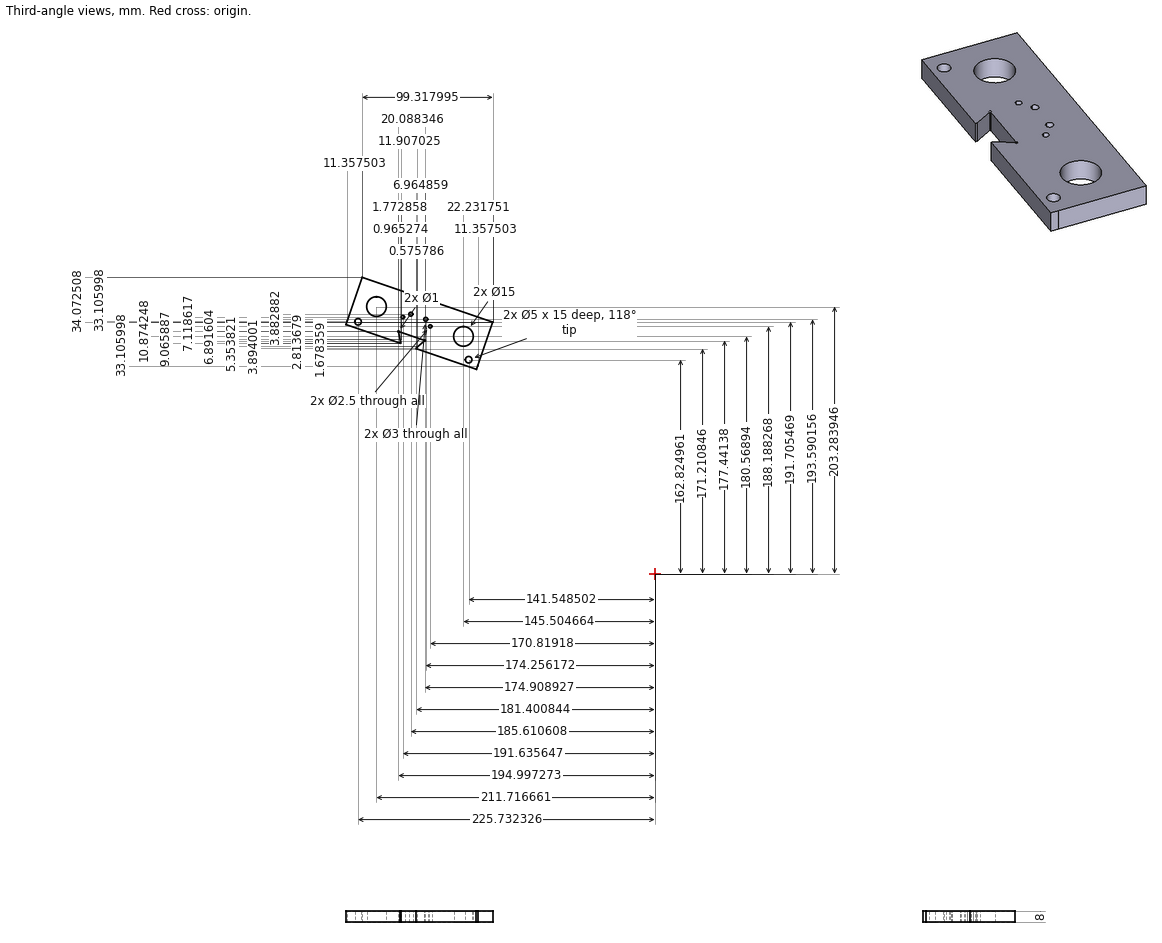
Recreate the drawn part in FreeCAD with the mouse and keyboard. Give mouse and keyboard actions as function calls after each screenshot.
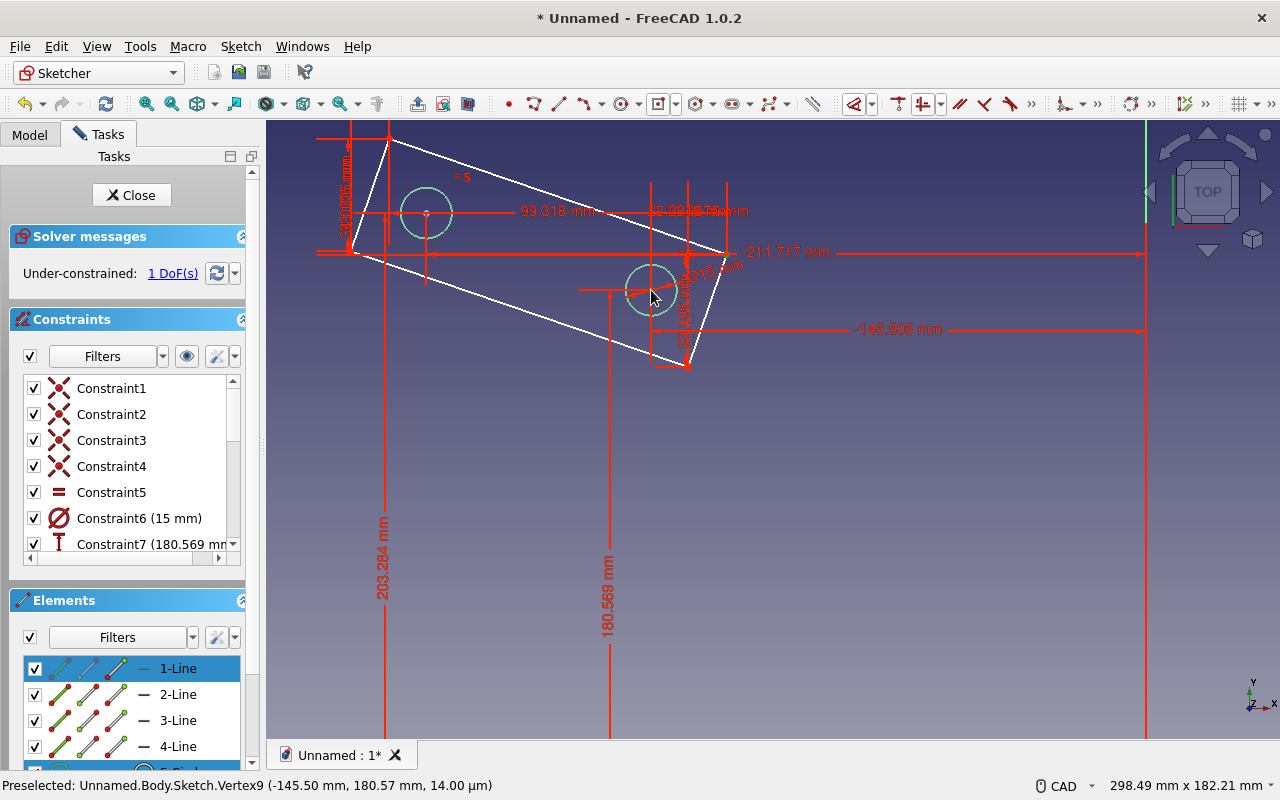
click(872, 104)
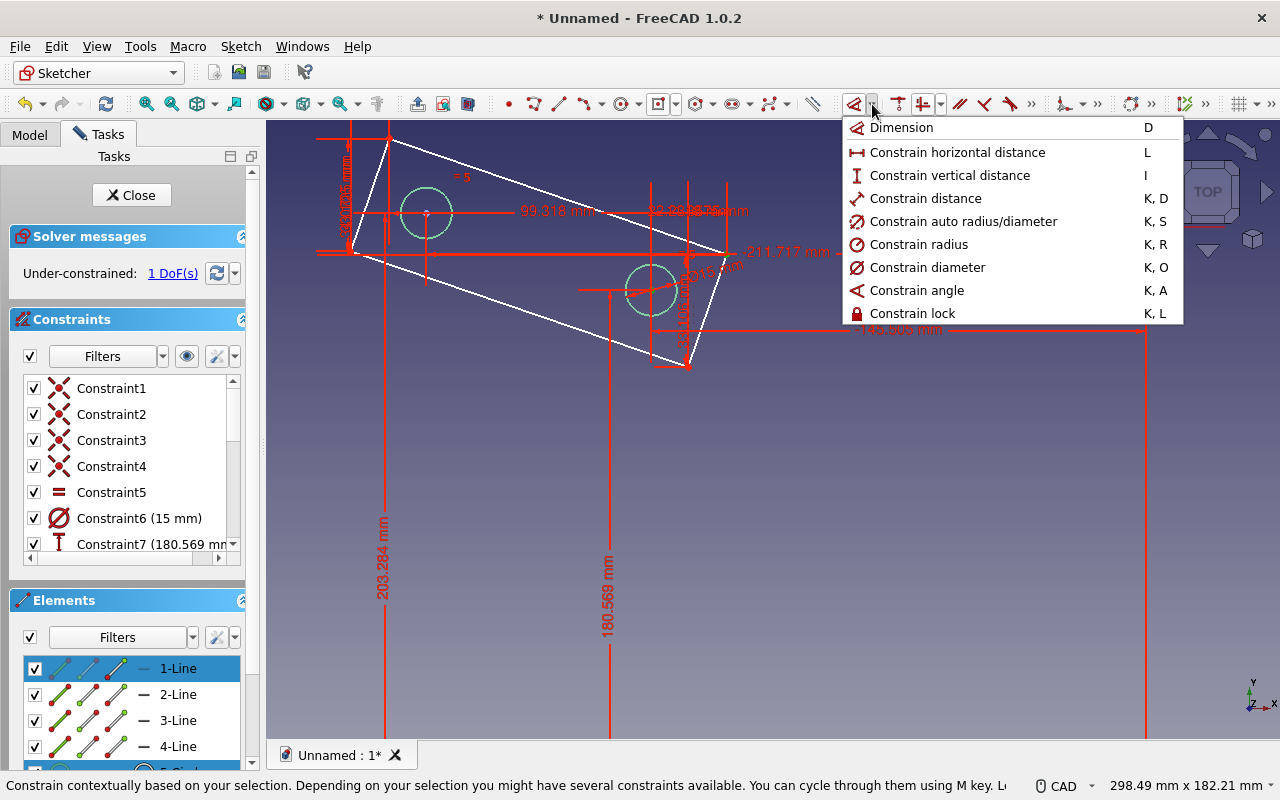
click(1013, 176)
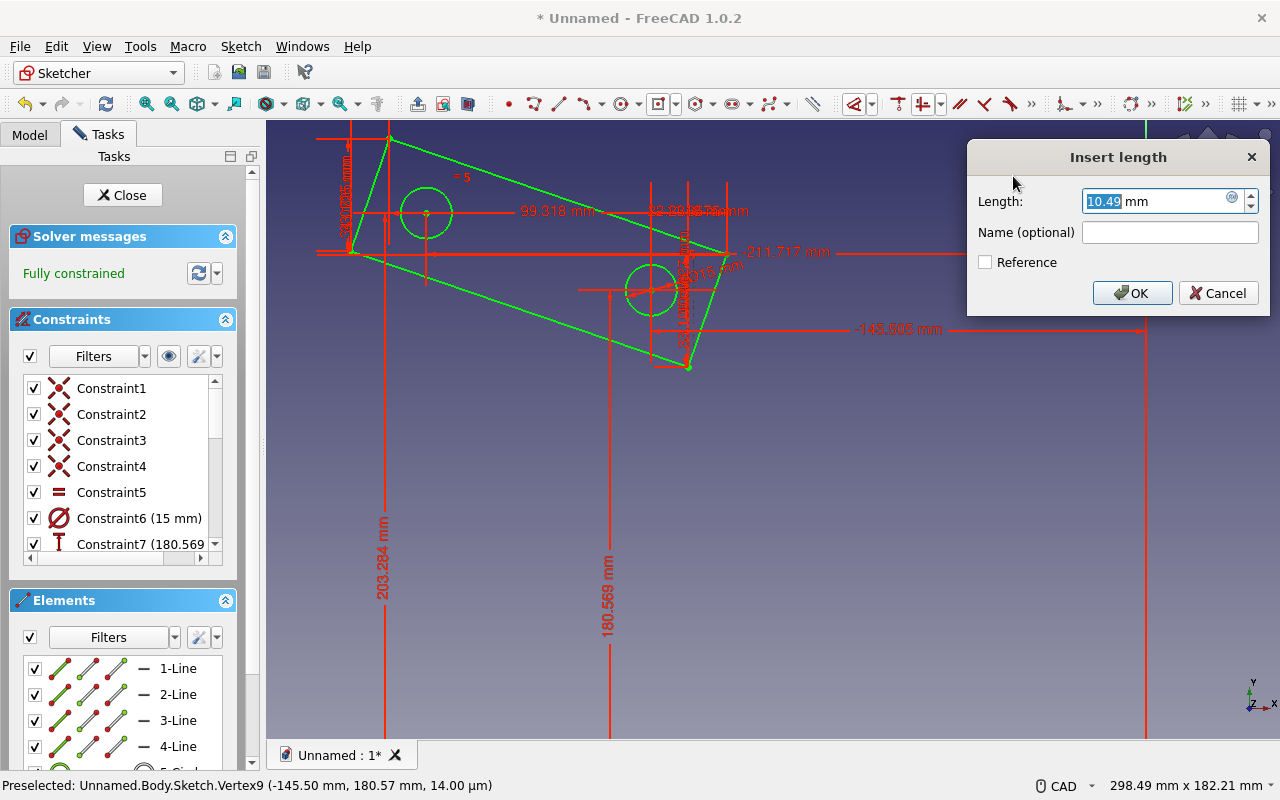
text(10.874248)
key(Return)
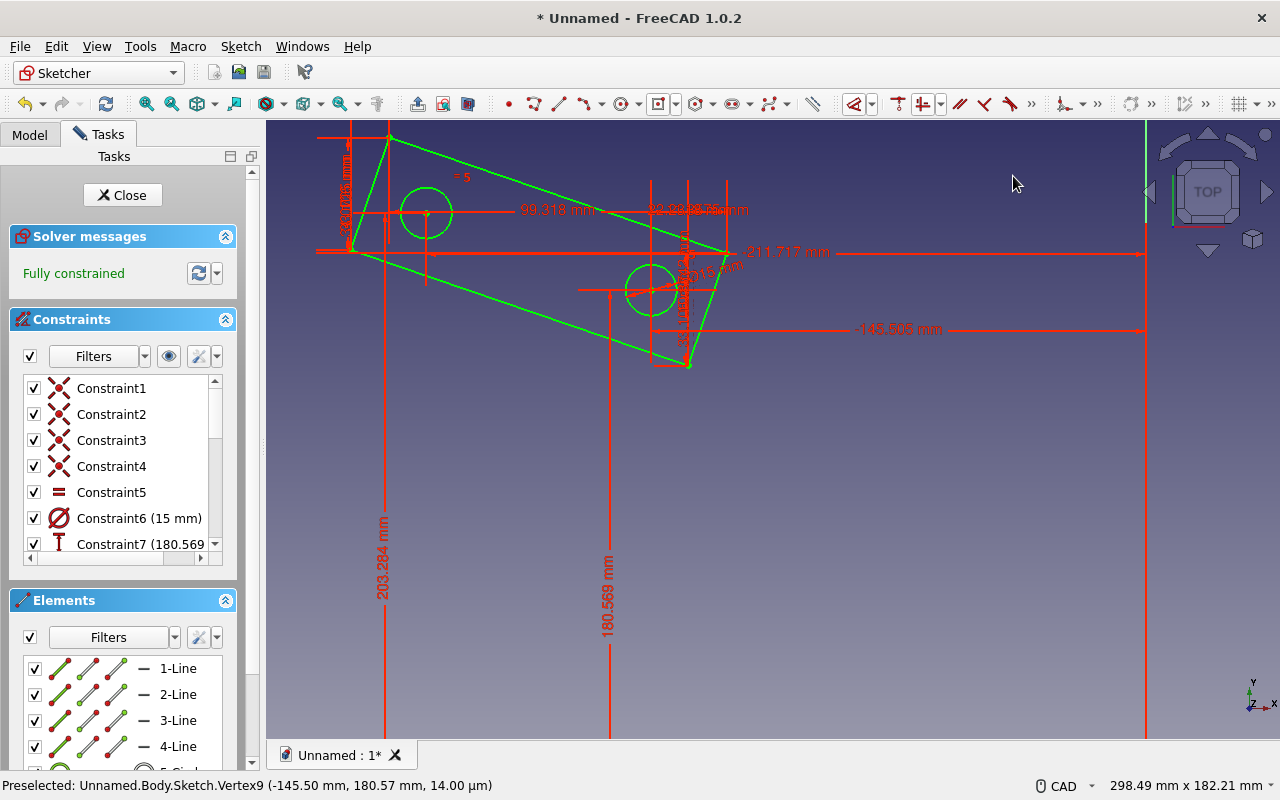
click(123, 195)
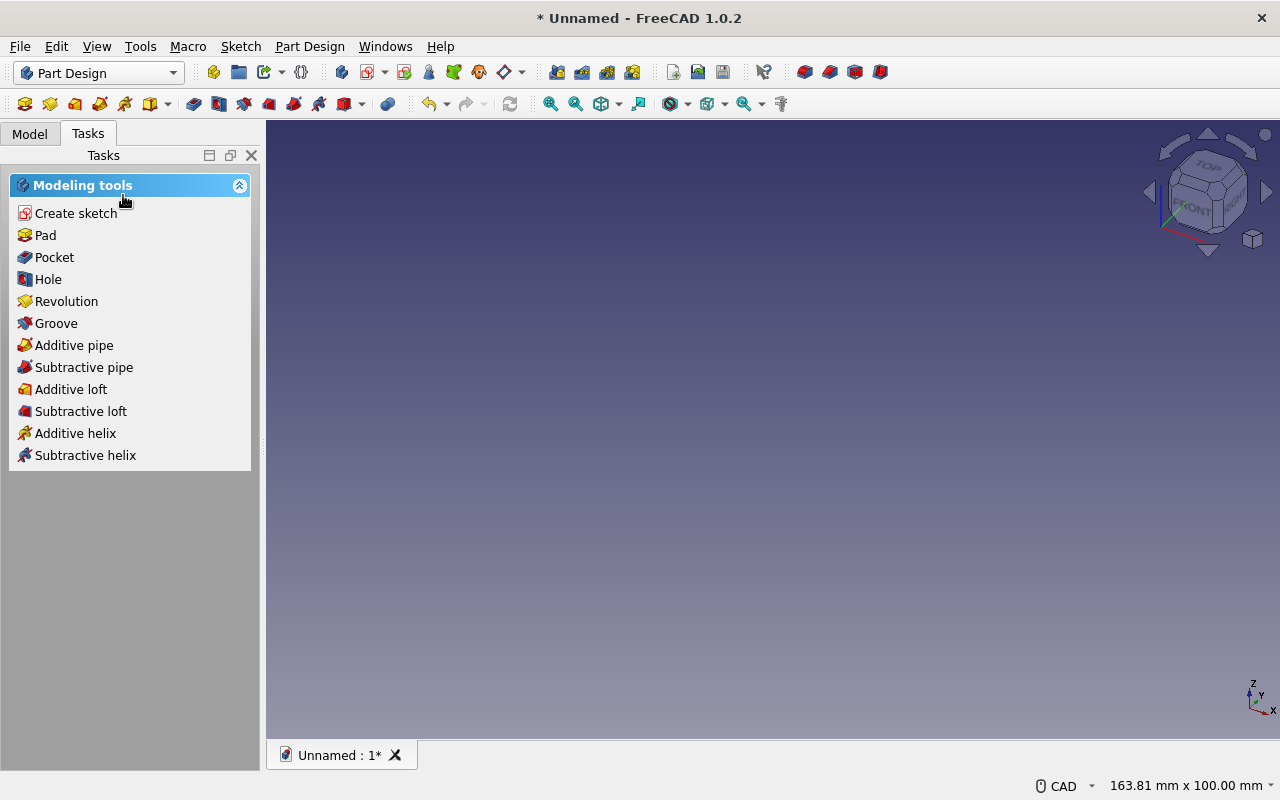
click(25, 104)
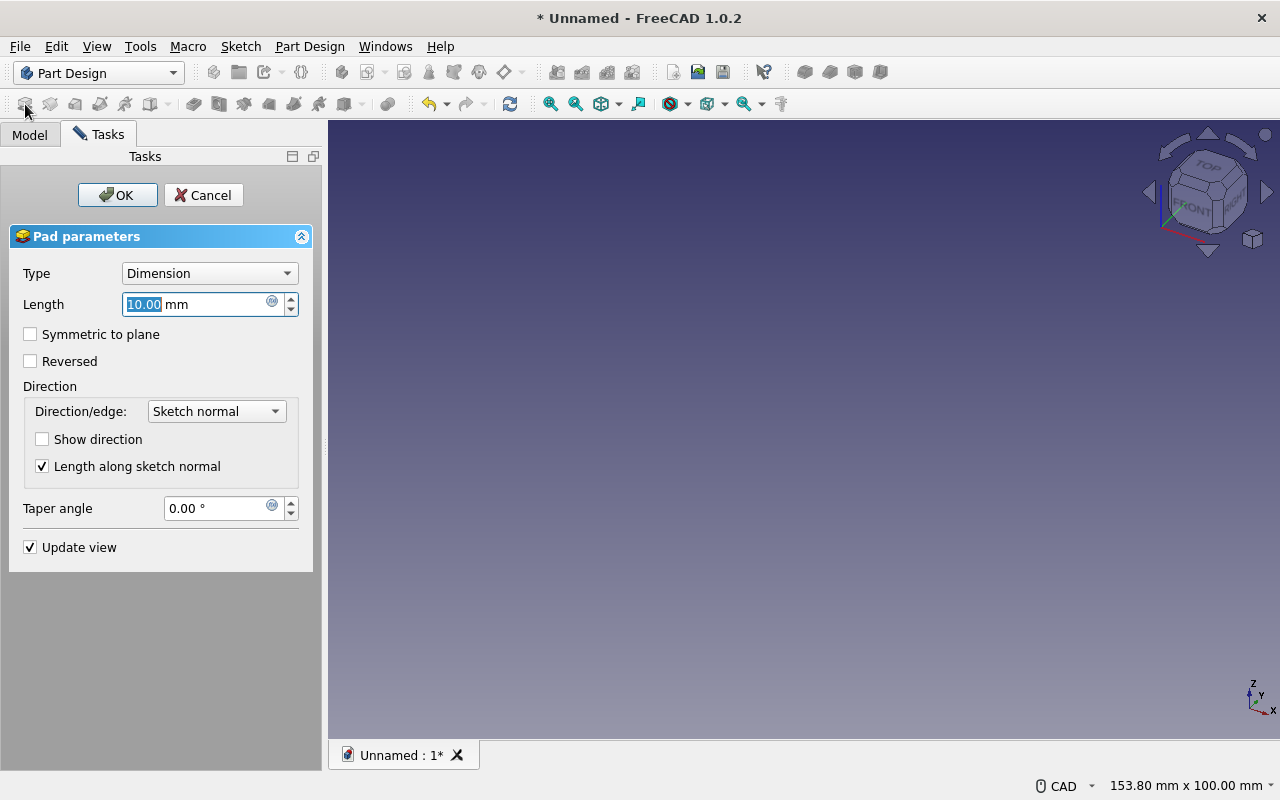
text(8)
key(Tab)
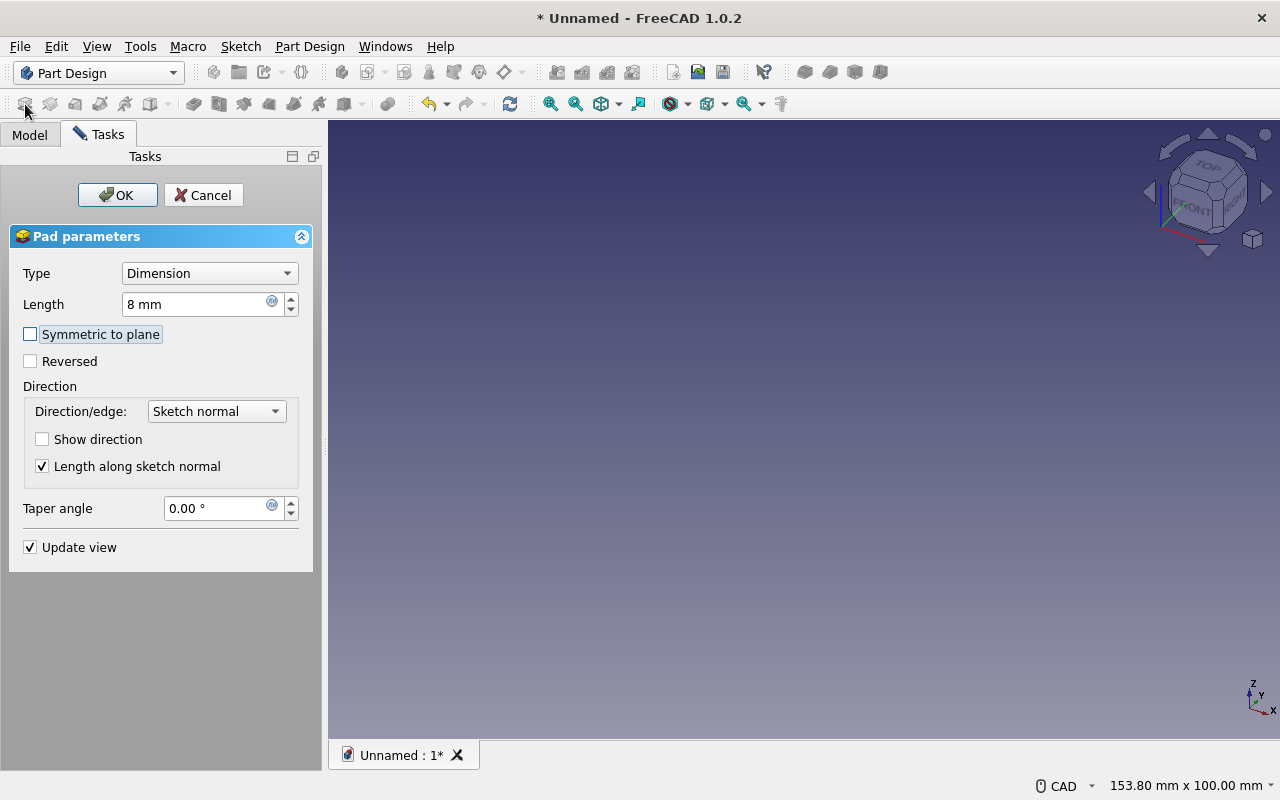
click(118, 195)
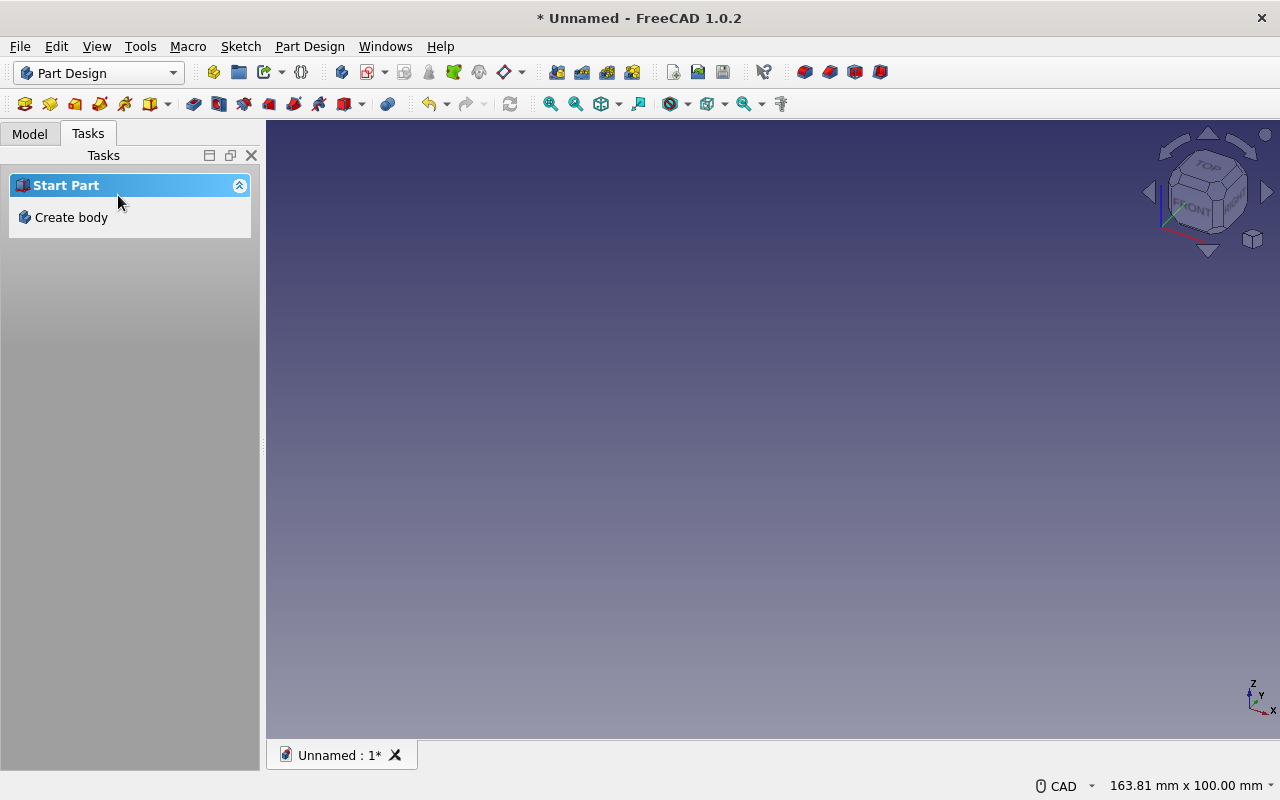
click(551, 104)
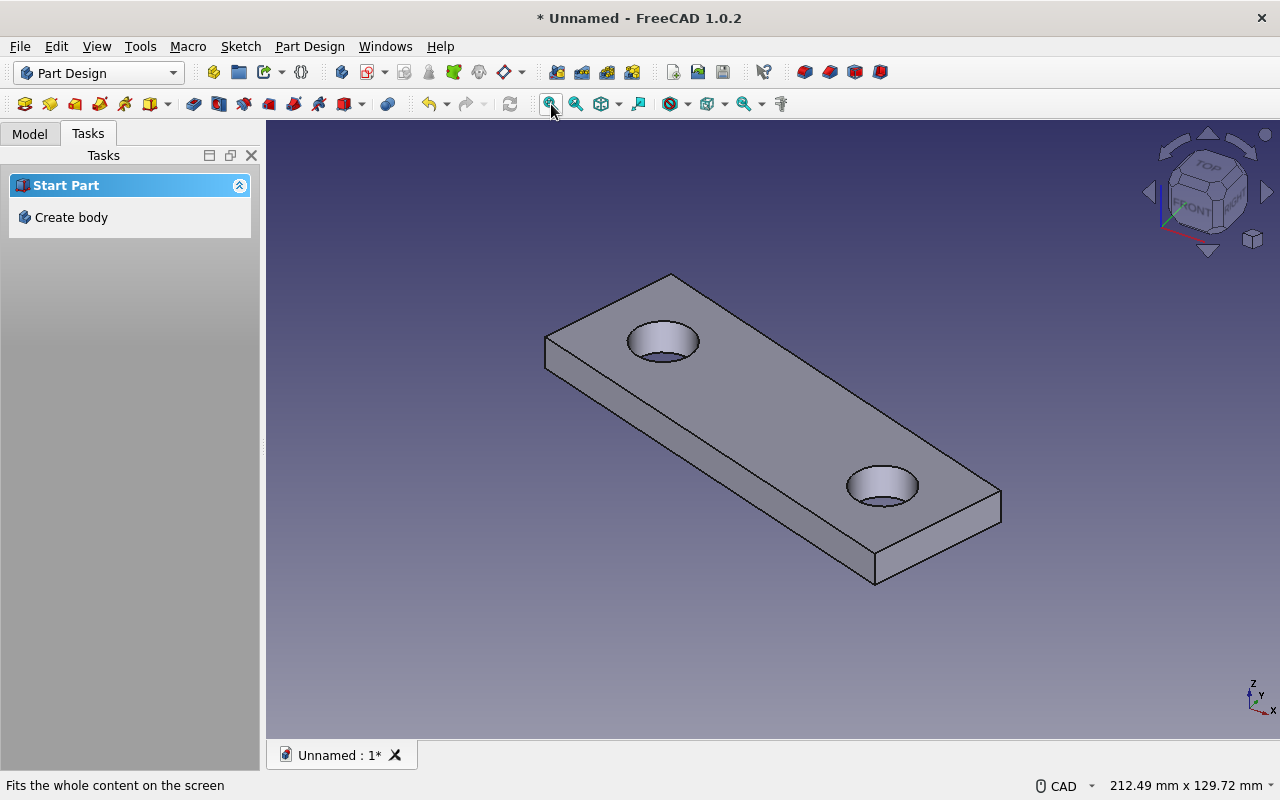
click(851, 553)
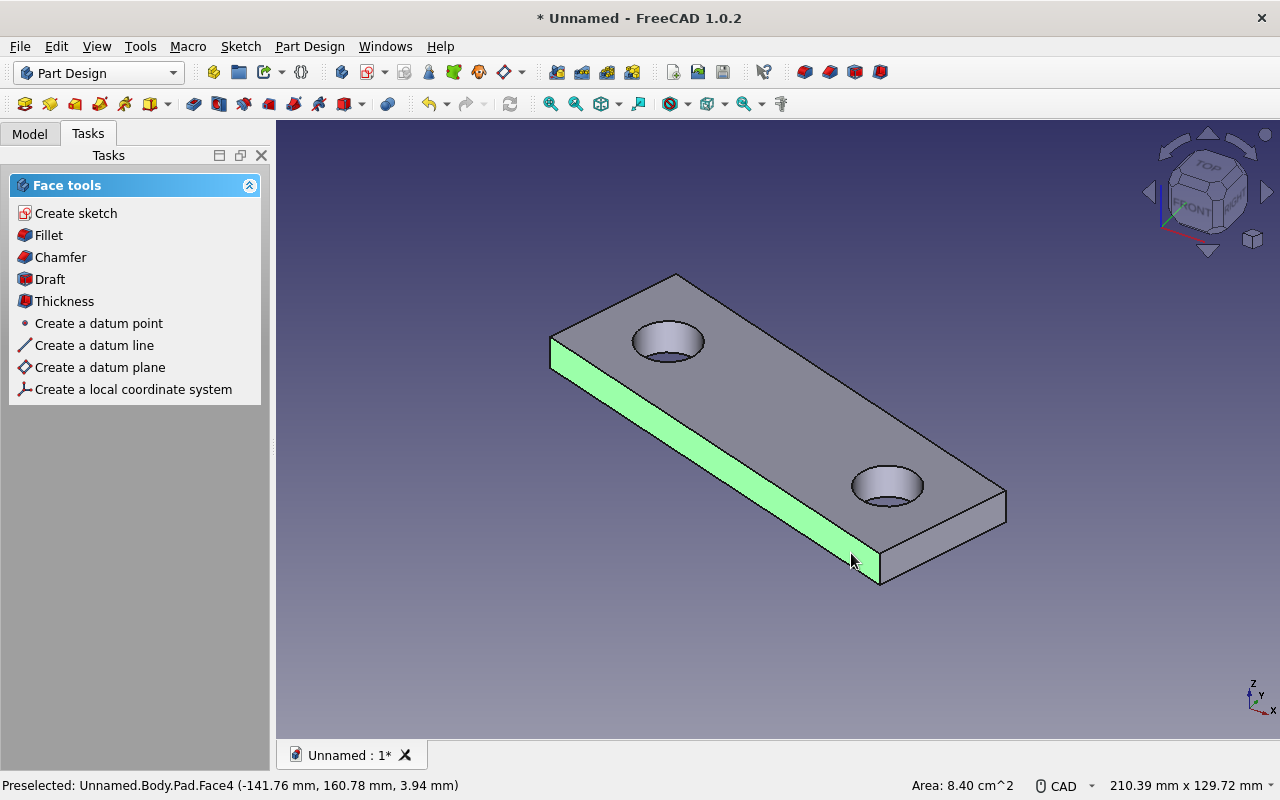
click(366, 72)